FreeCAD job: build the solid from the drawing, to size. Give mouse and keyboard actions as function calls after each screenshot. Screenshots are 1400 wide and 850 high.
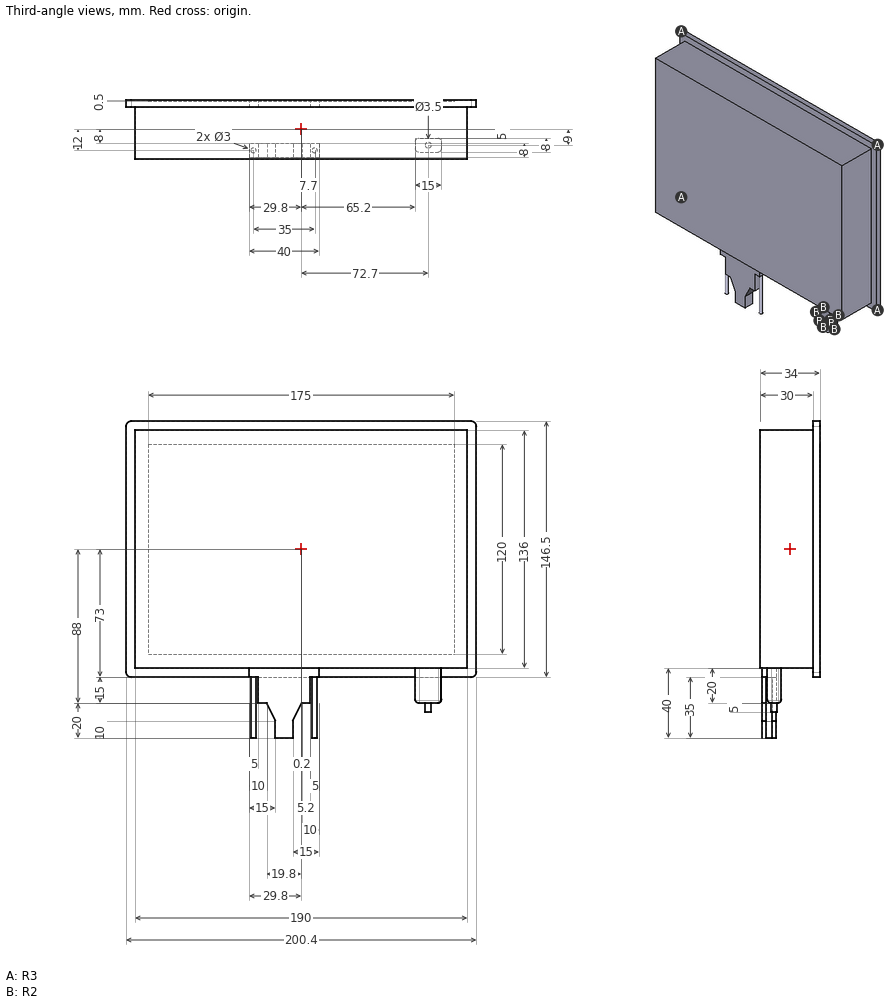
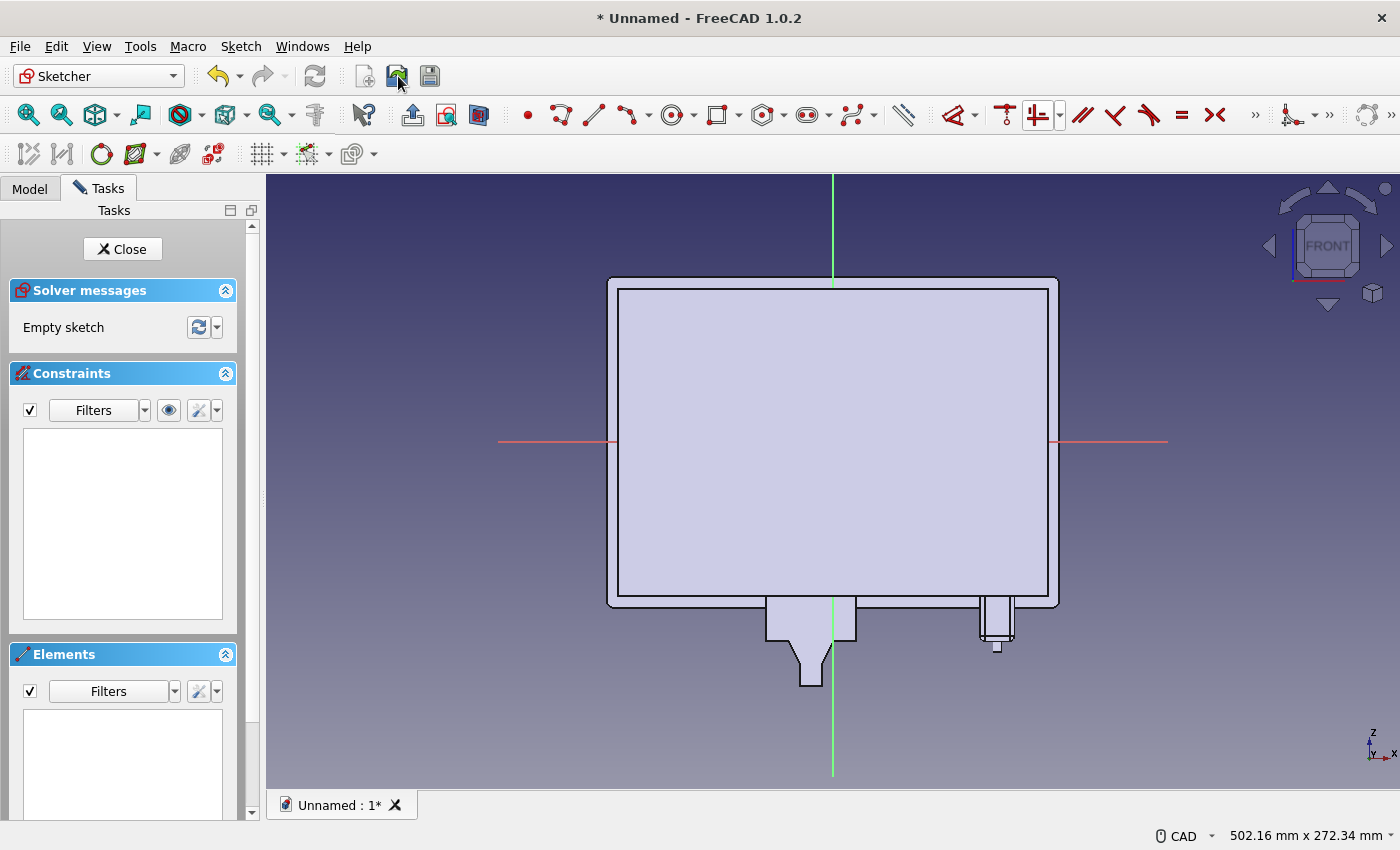
scroll(867, 615, up, 3)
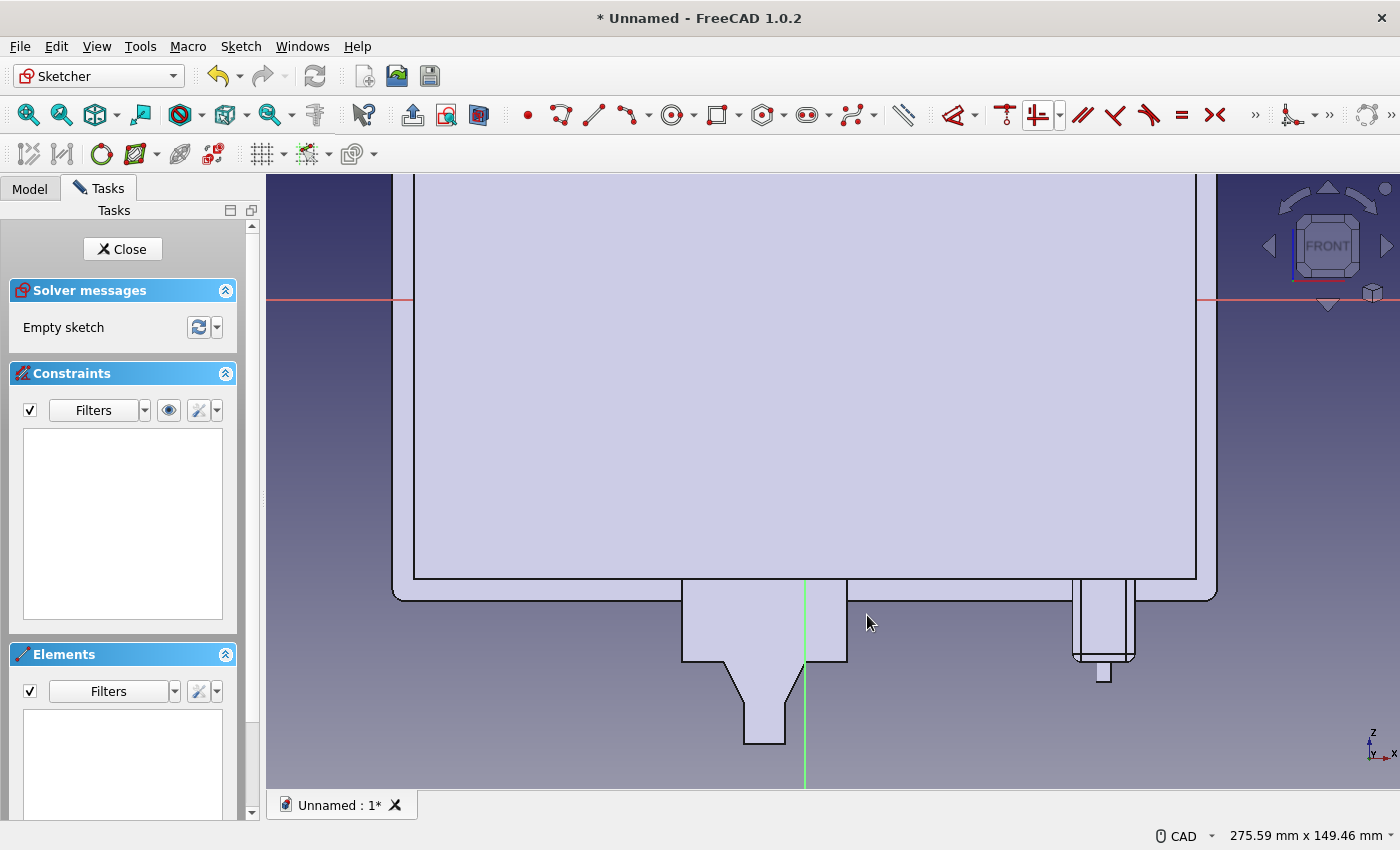
click(716, 116)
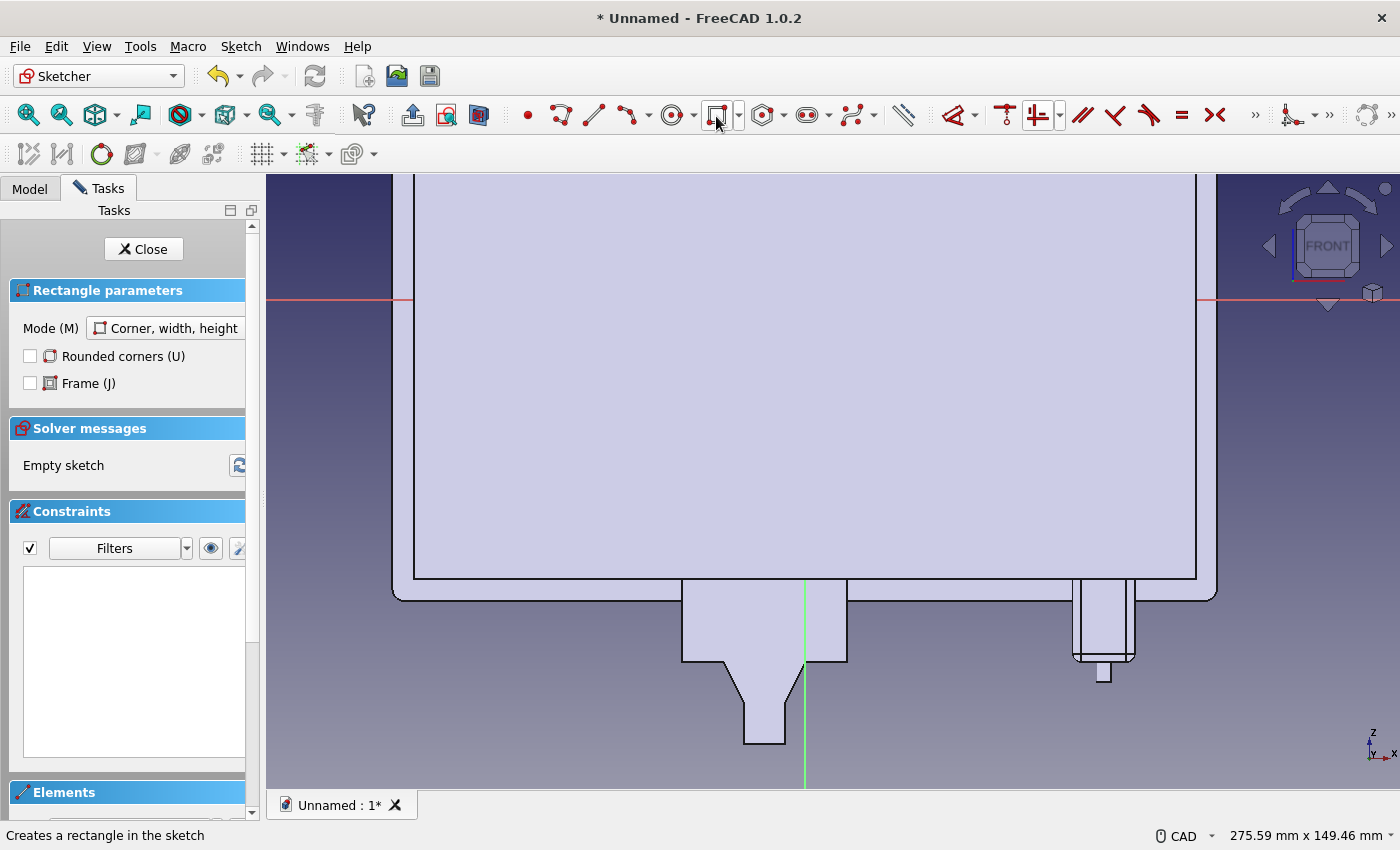
click(682, 600)
move(703, 662)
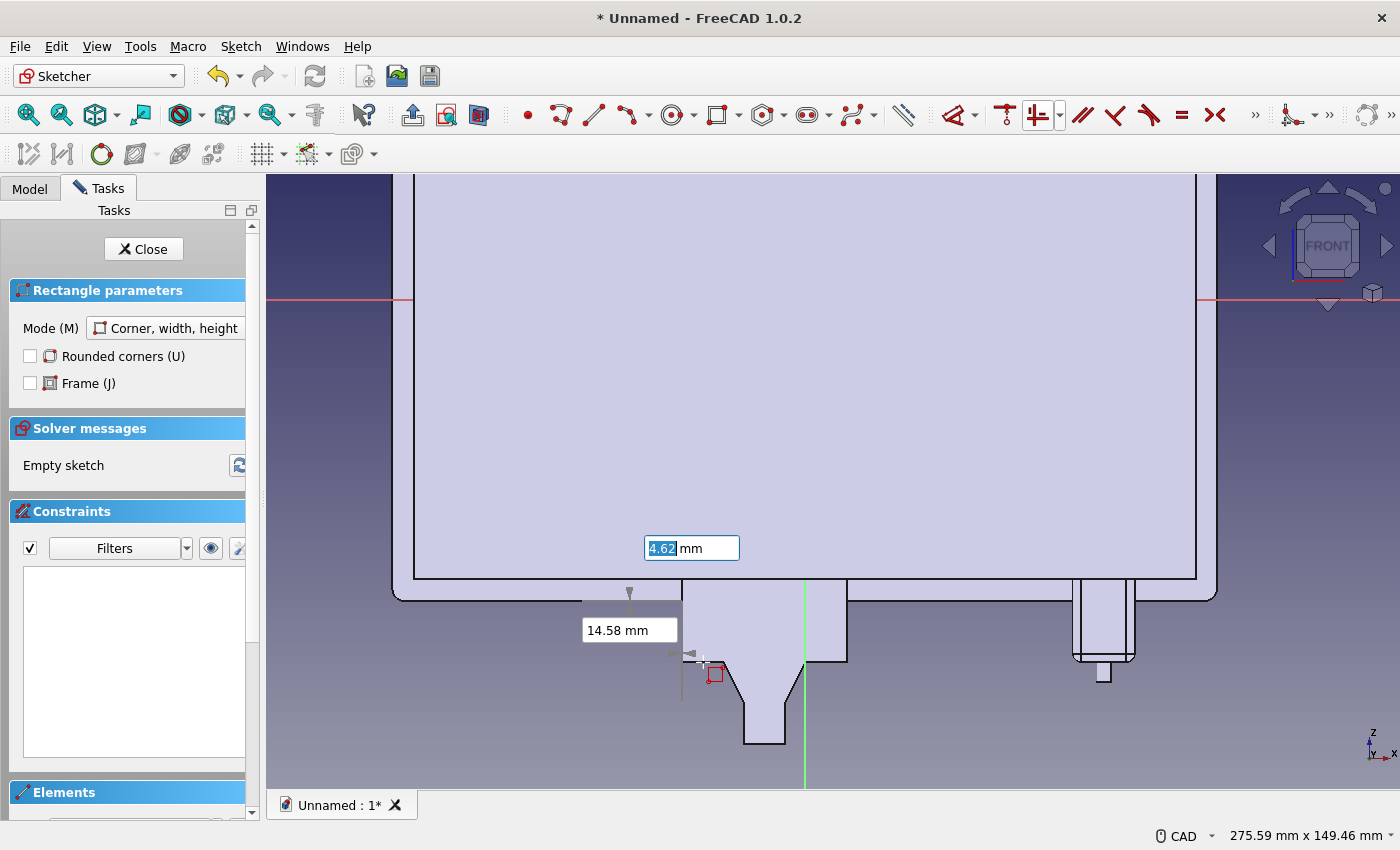
text(5)
key(Tab)
text(15)
key(Return)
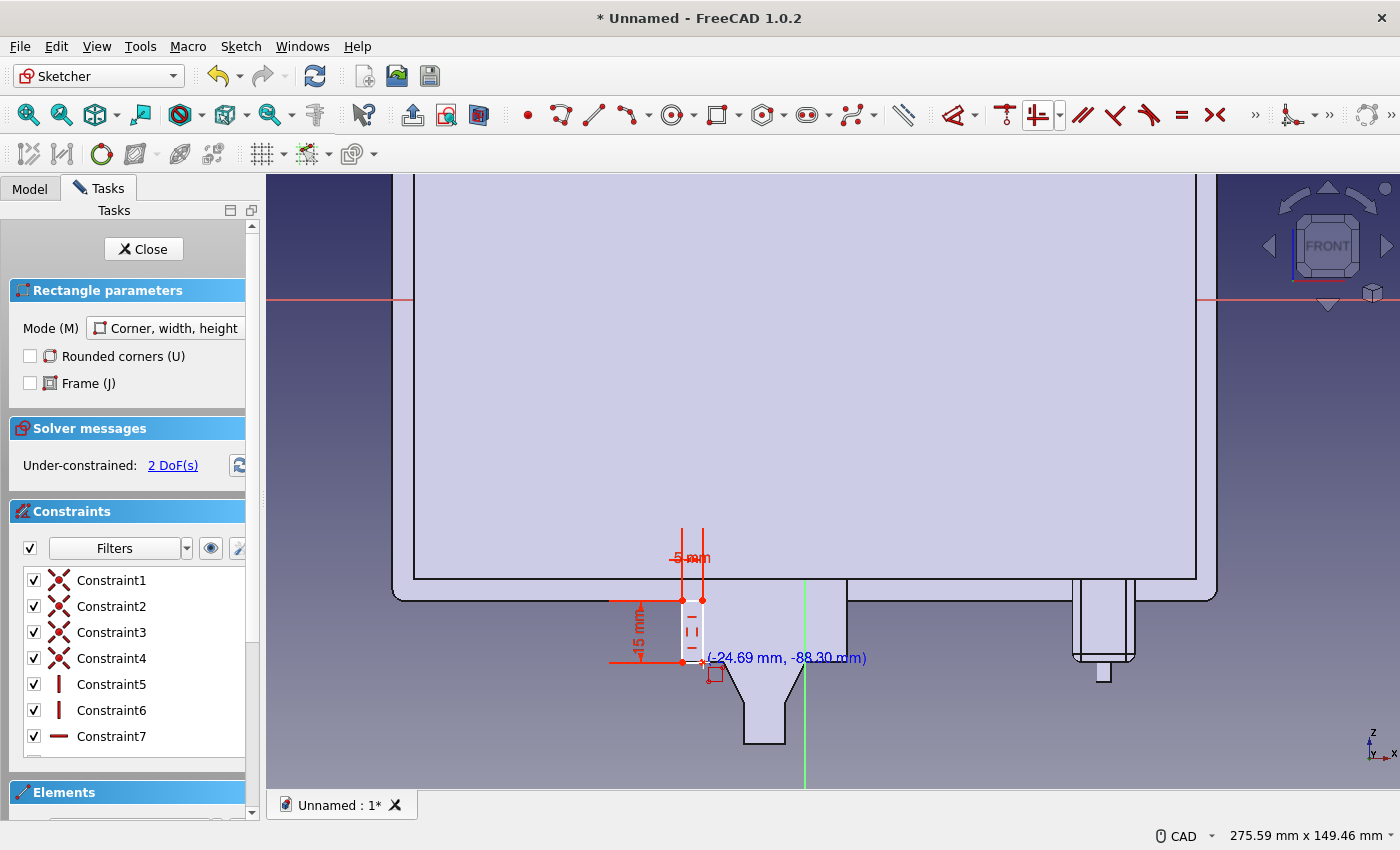
click(826, 600)
move(847, 662)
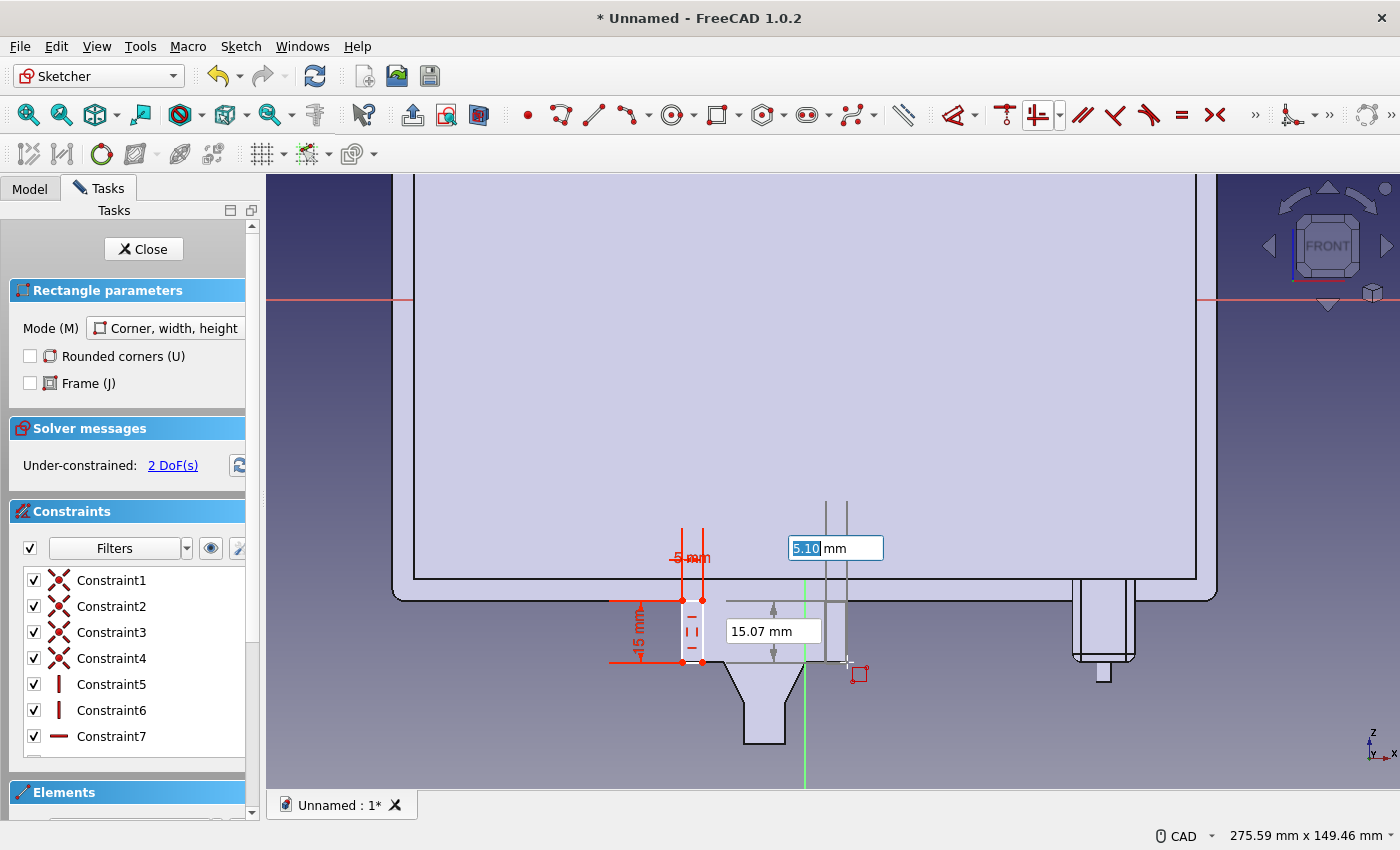
text(5)
key(Tab)
text(15)
key(Return)
key(Escape)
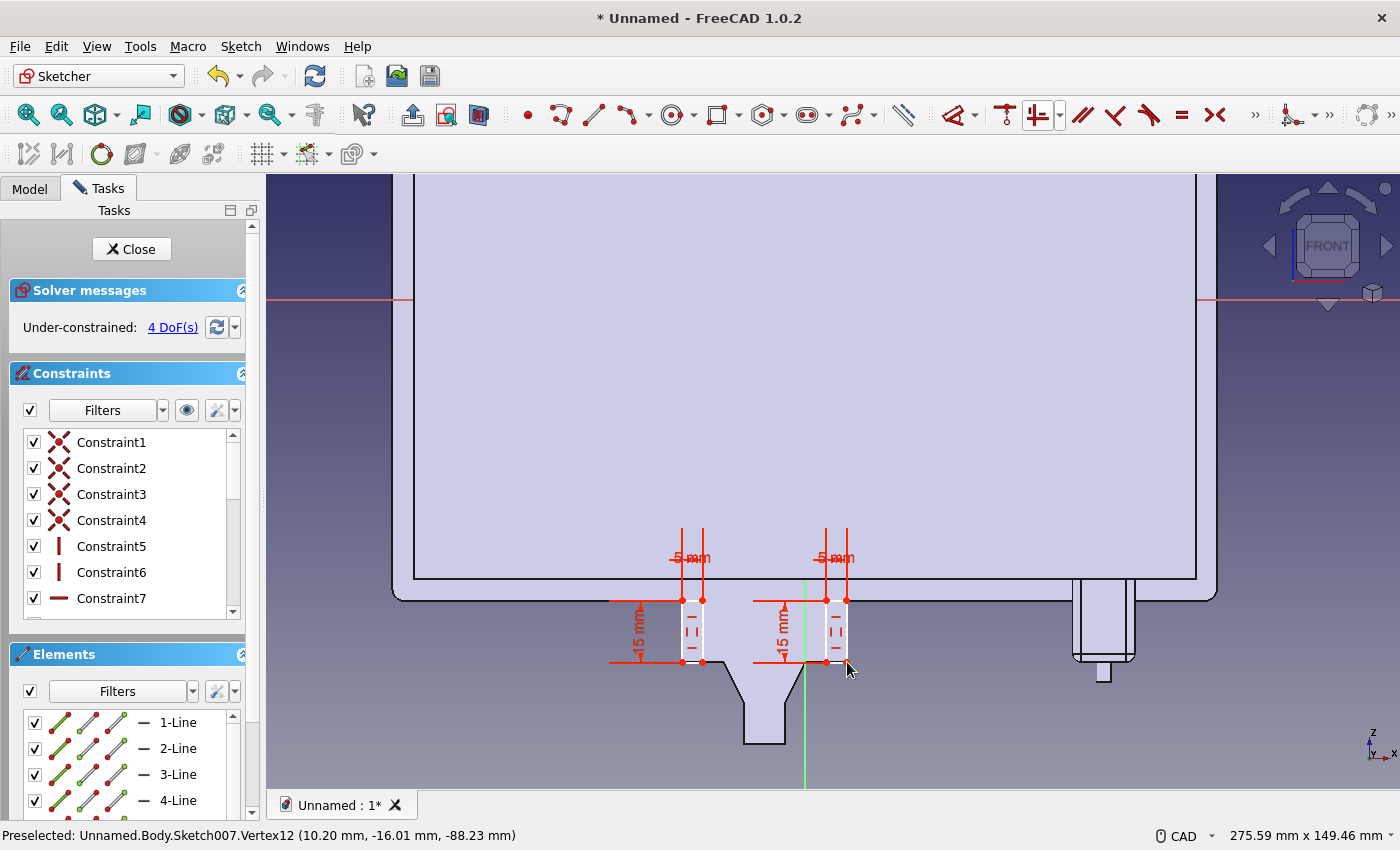
click(952, 116)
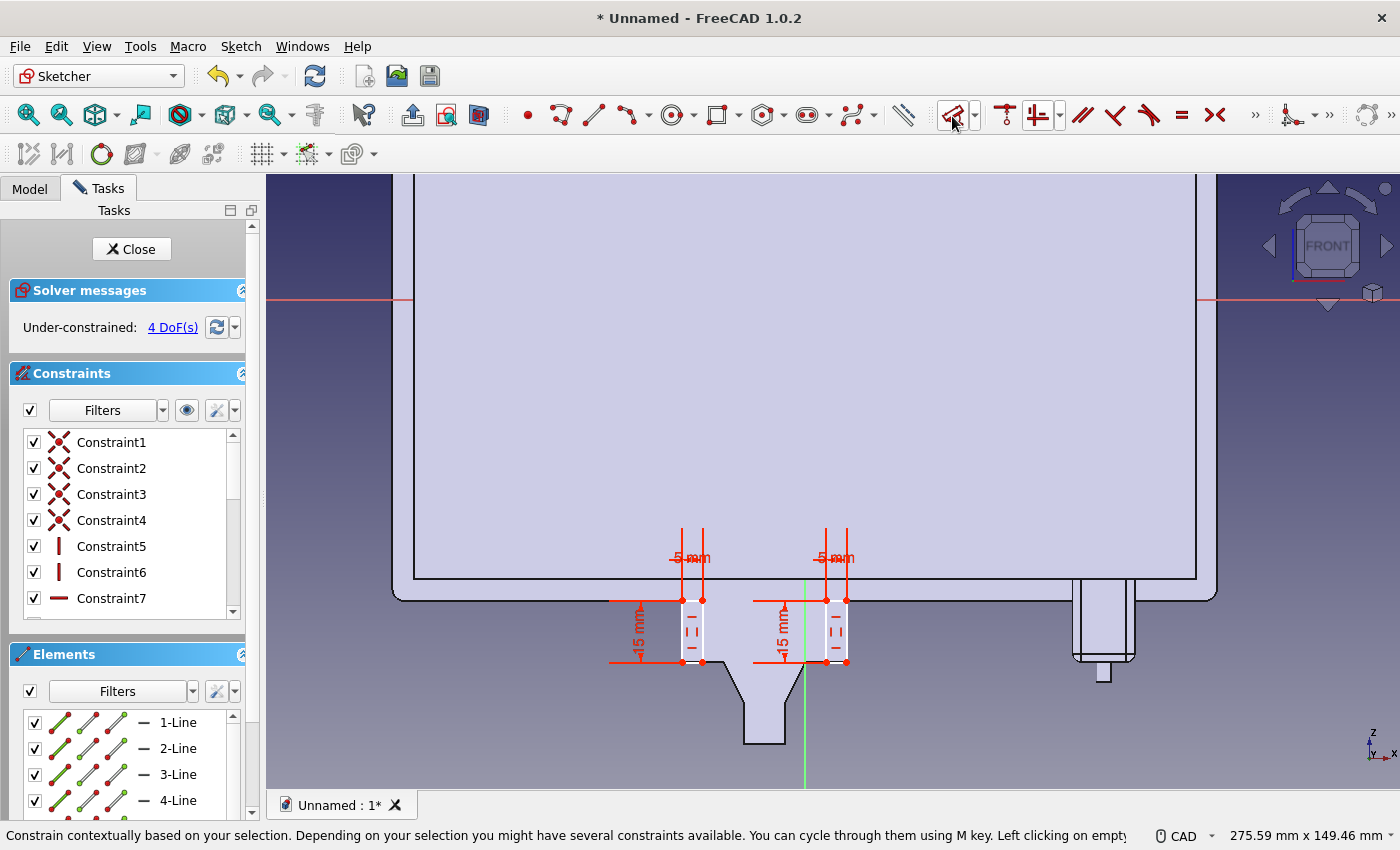
click(682, 601)
click(648, 450)